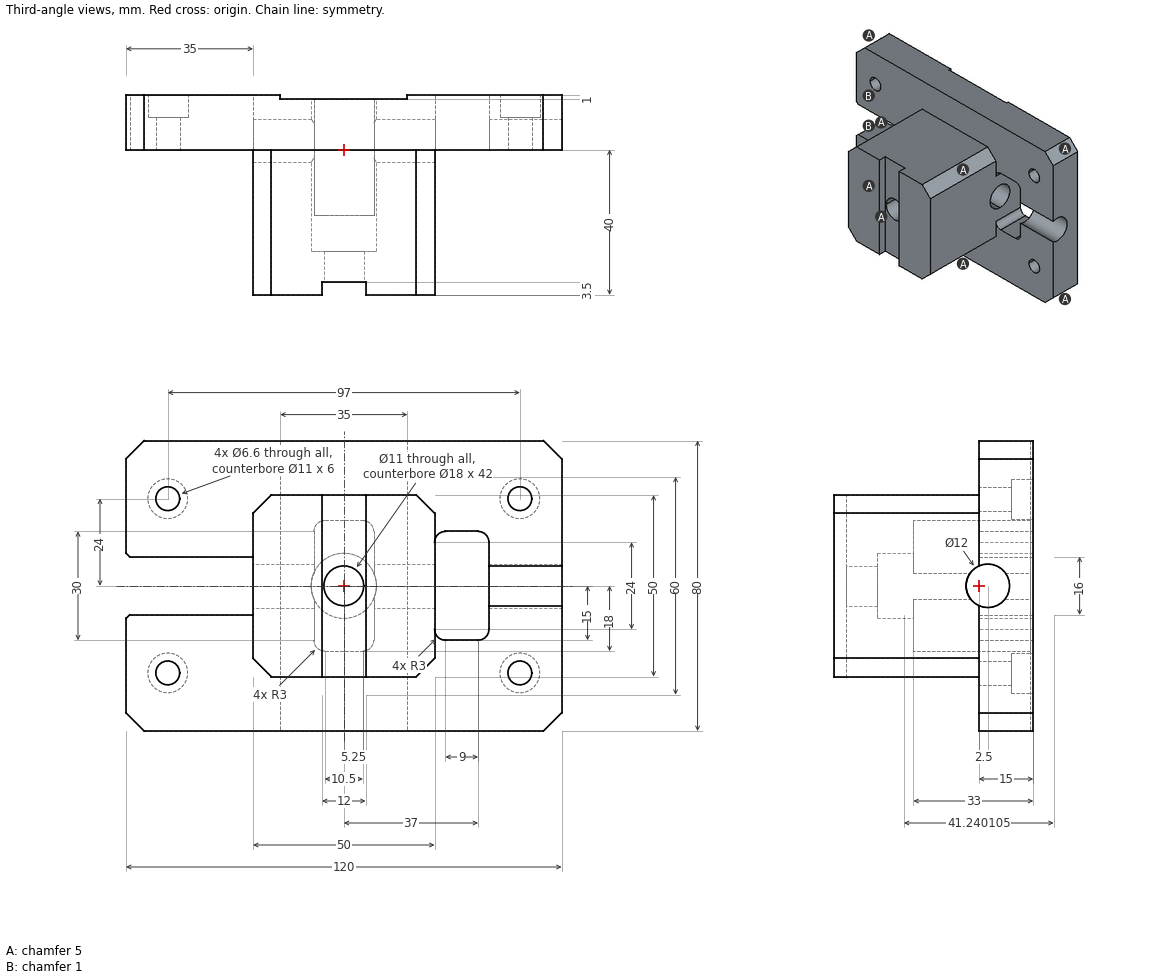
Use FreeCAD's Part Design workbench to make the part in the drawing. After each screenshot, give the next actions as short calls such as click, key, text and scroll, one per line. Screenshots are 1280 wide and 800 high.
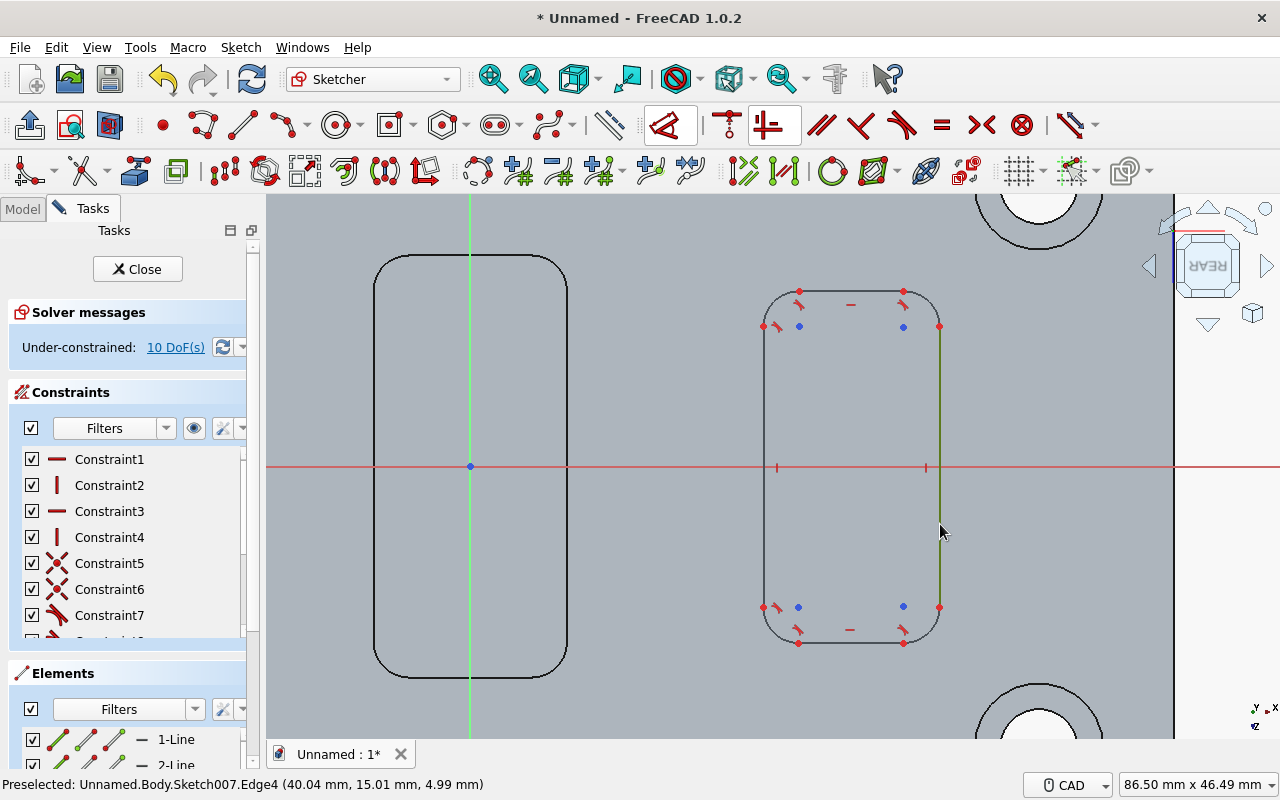
click(919, 639)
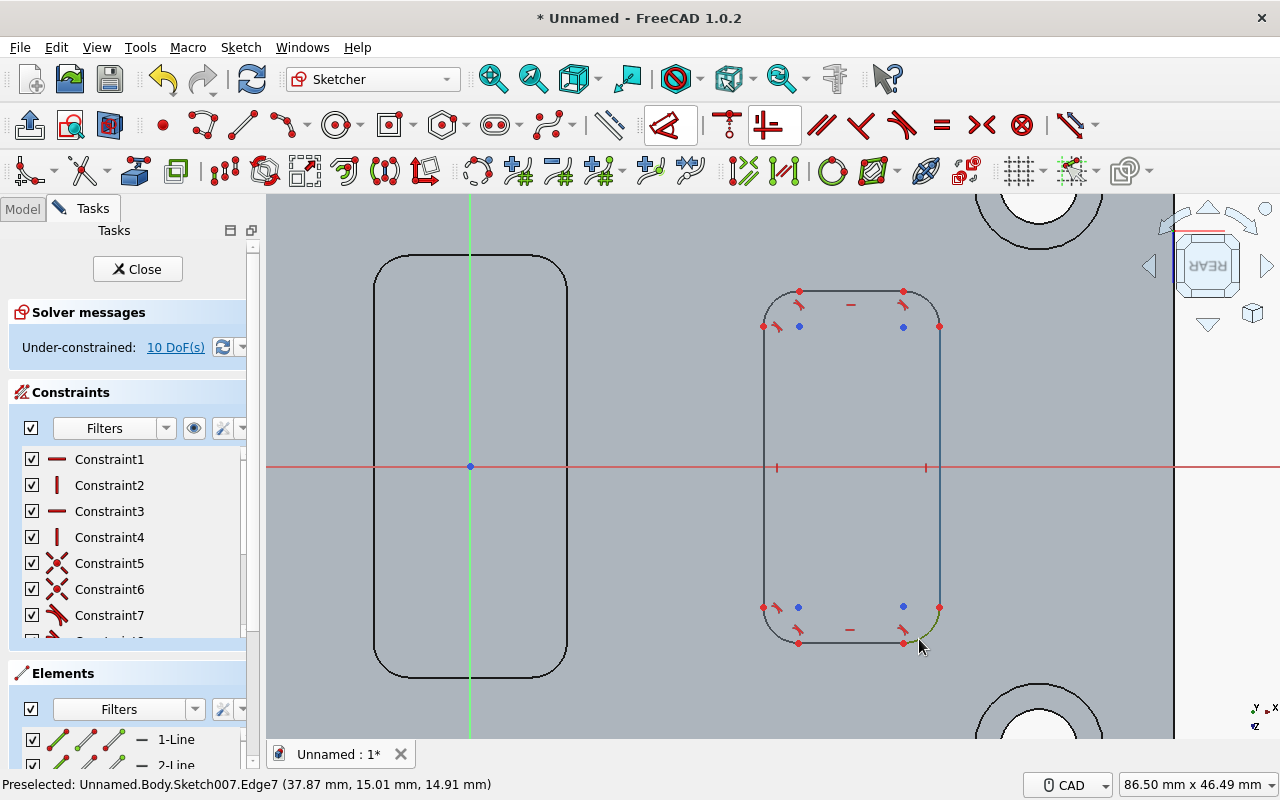
click(902, 126)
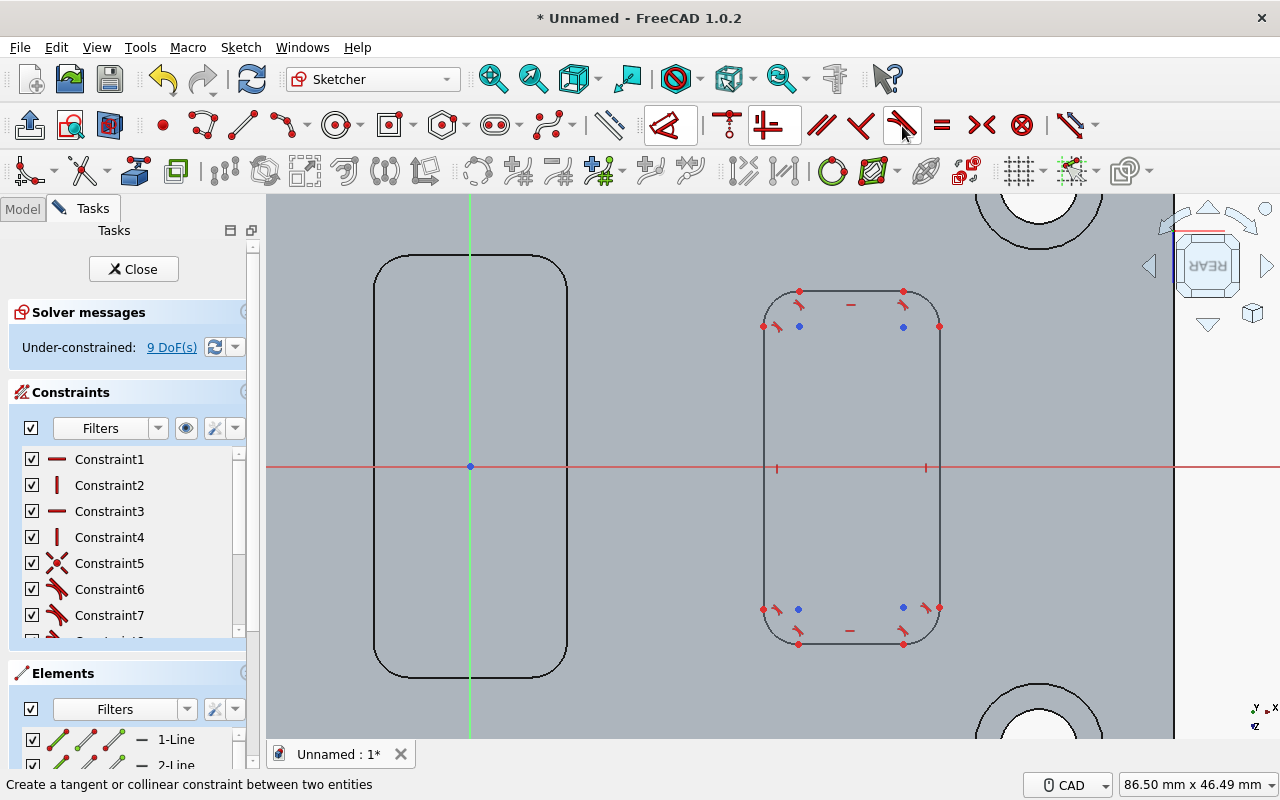
click(940, 524)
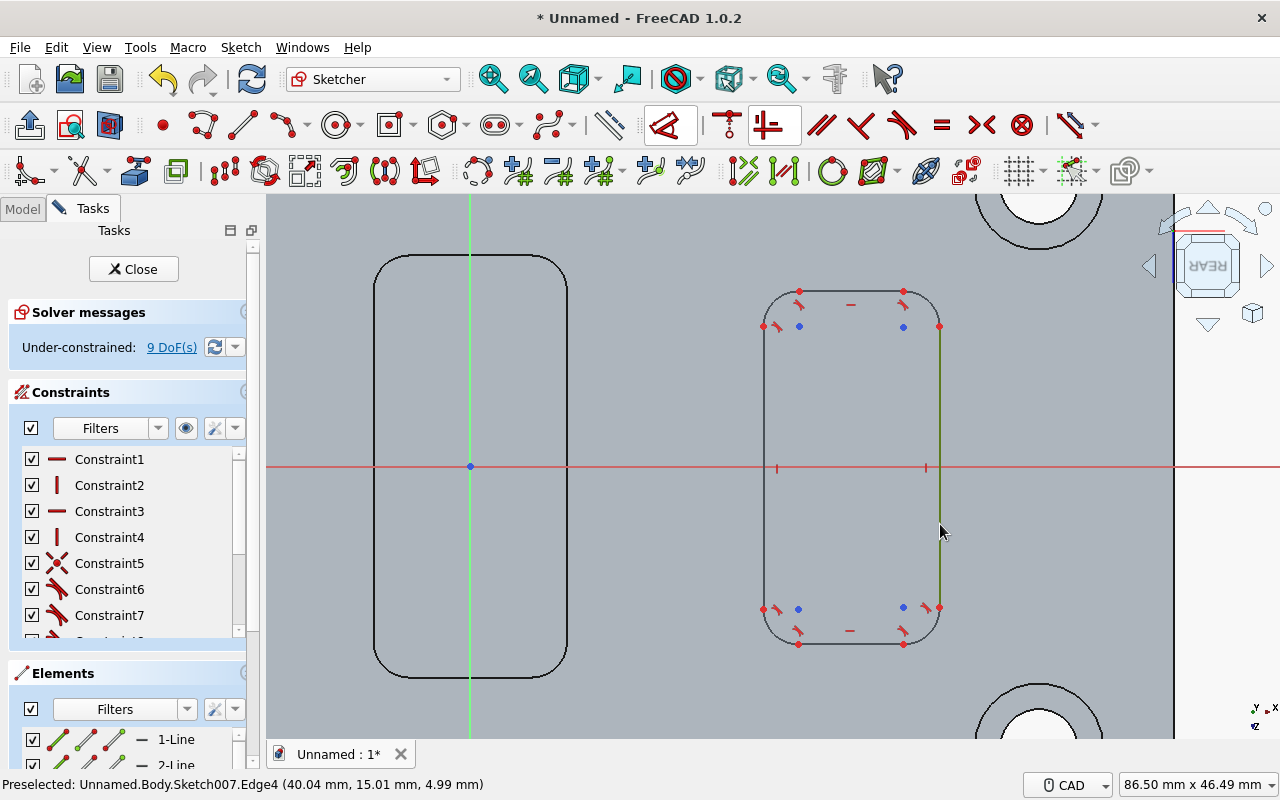
click(936, 311)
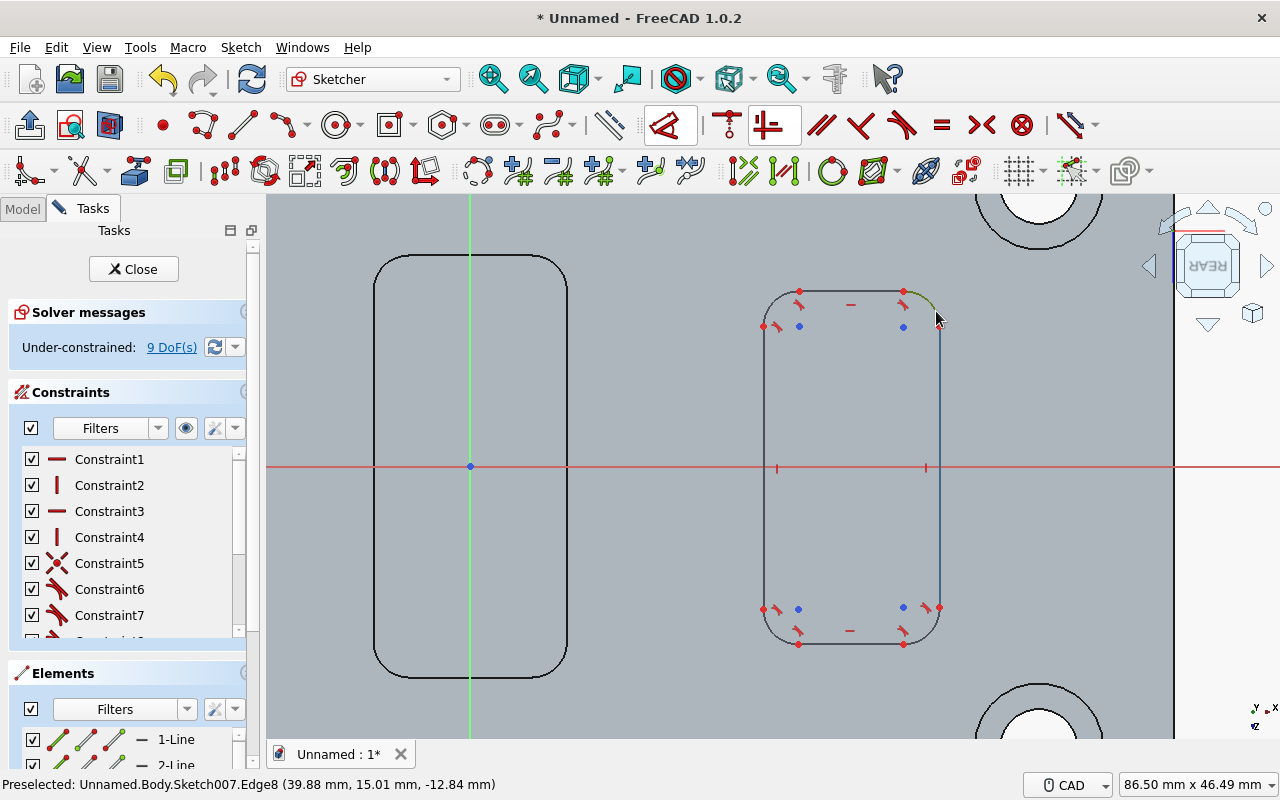
click(902, 126)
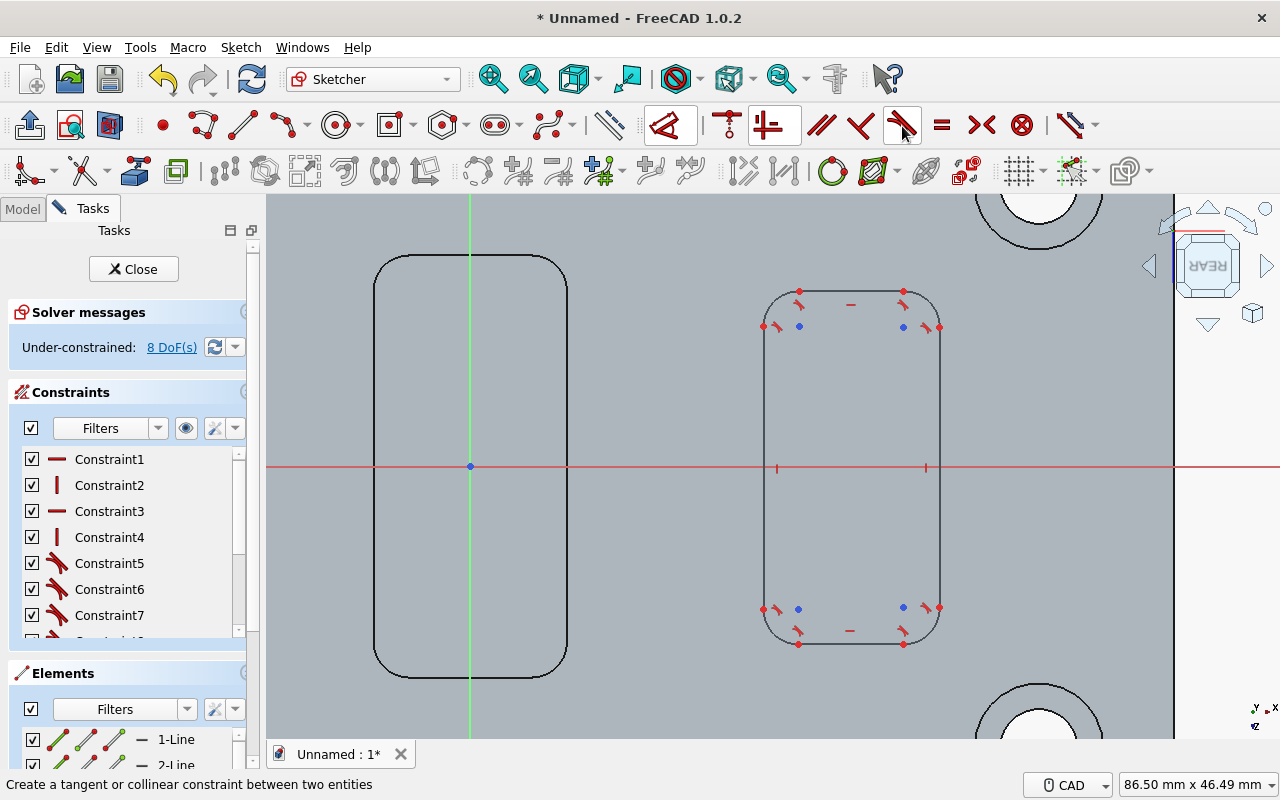
click(783, 295)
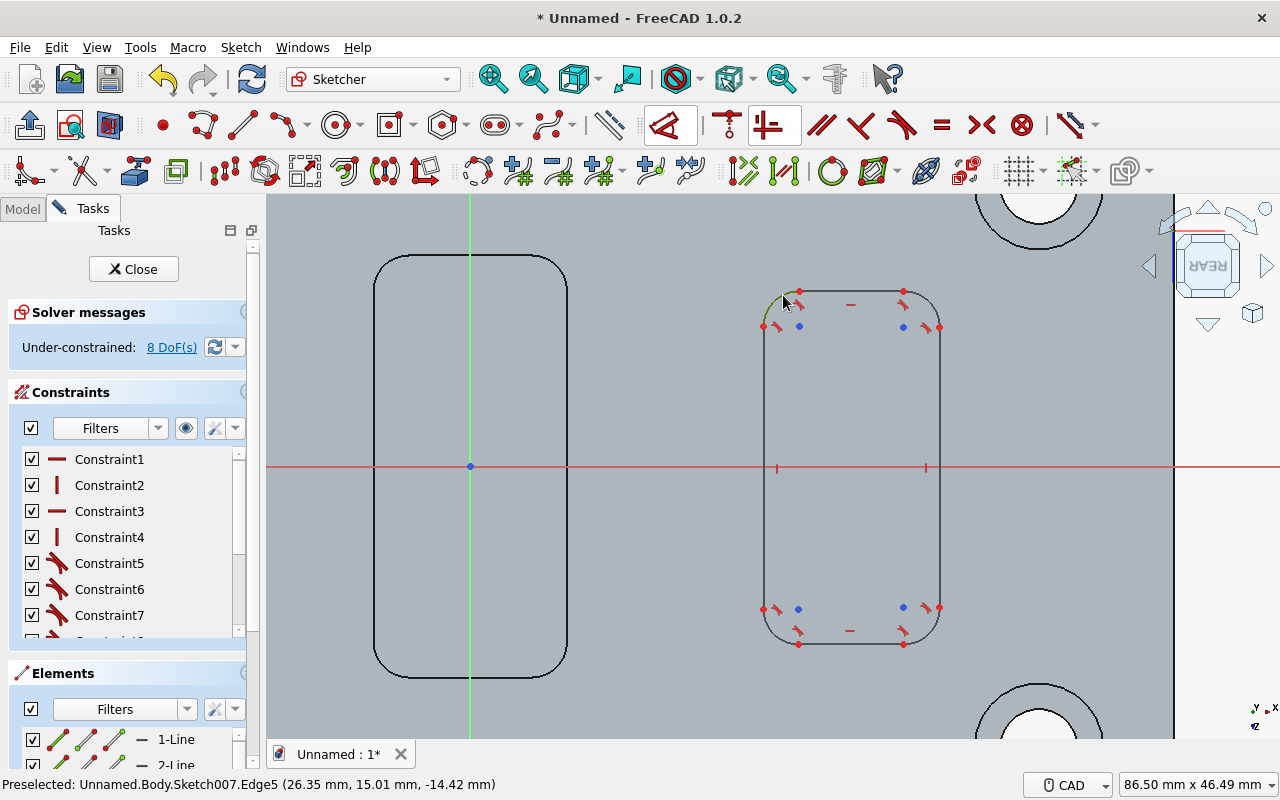
click(767, 625)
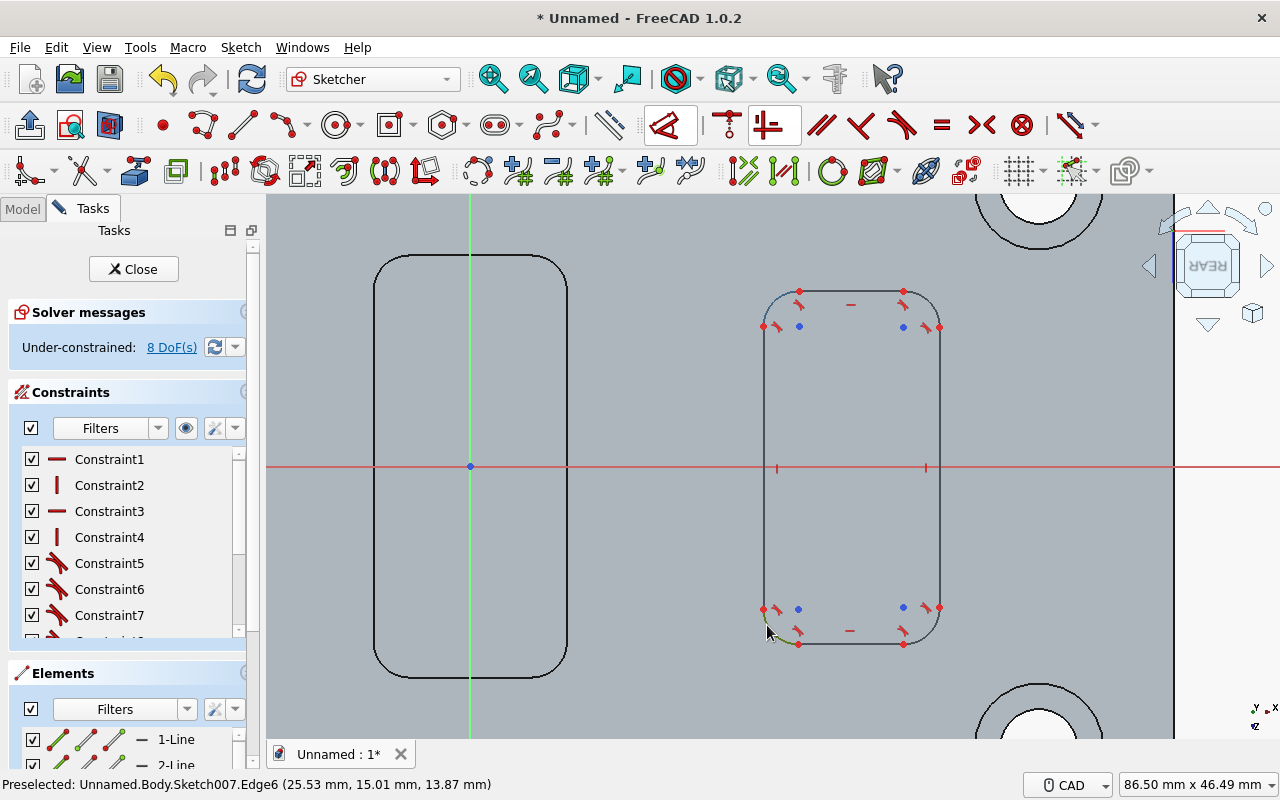
click(920, 640)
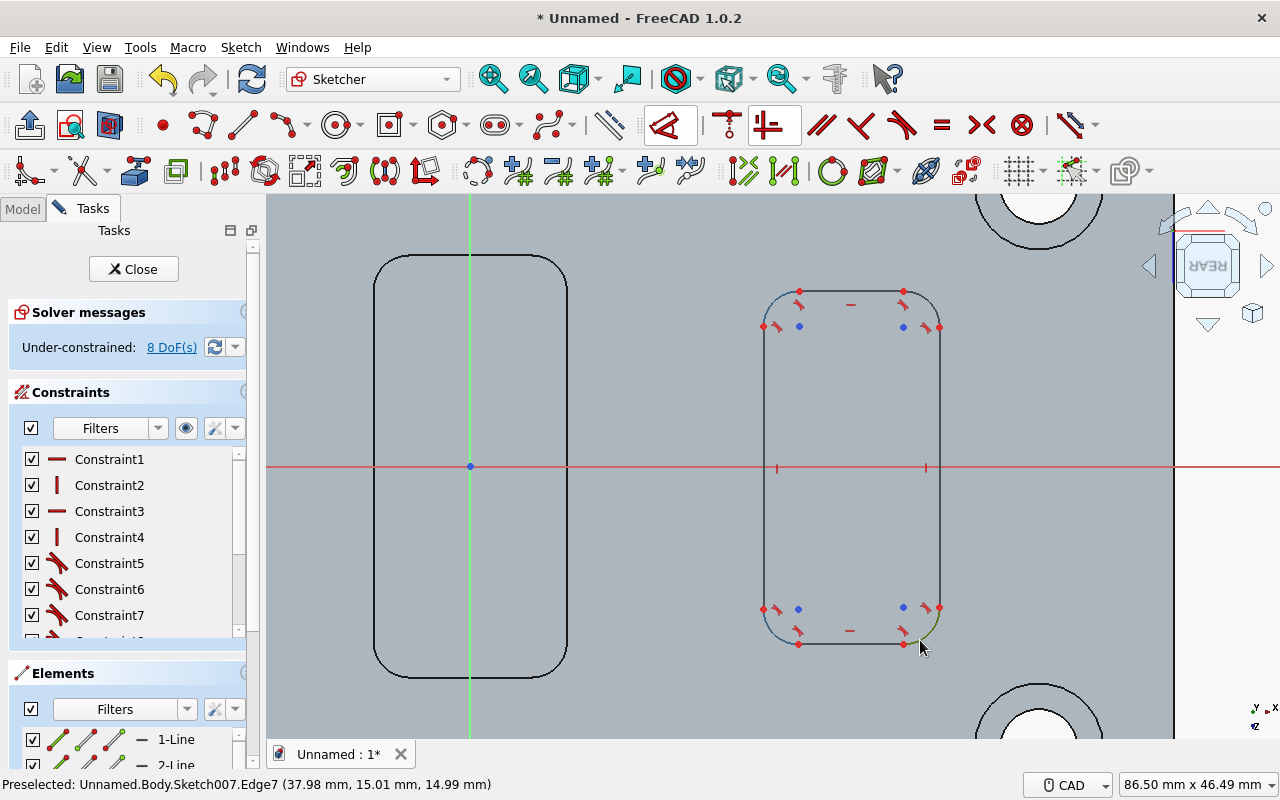
click(936, 311)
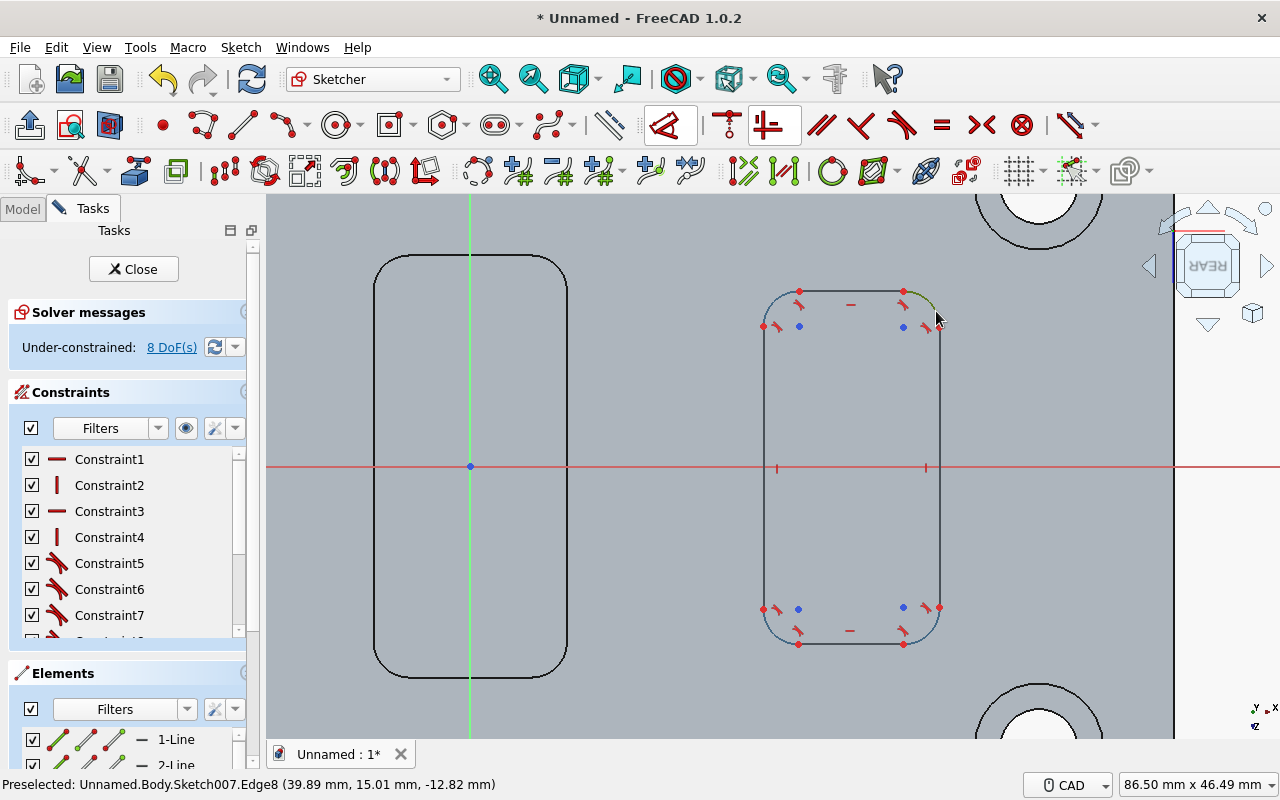
click(942, 126)